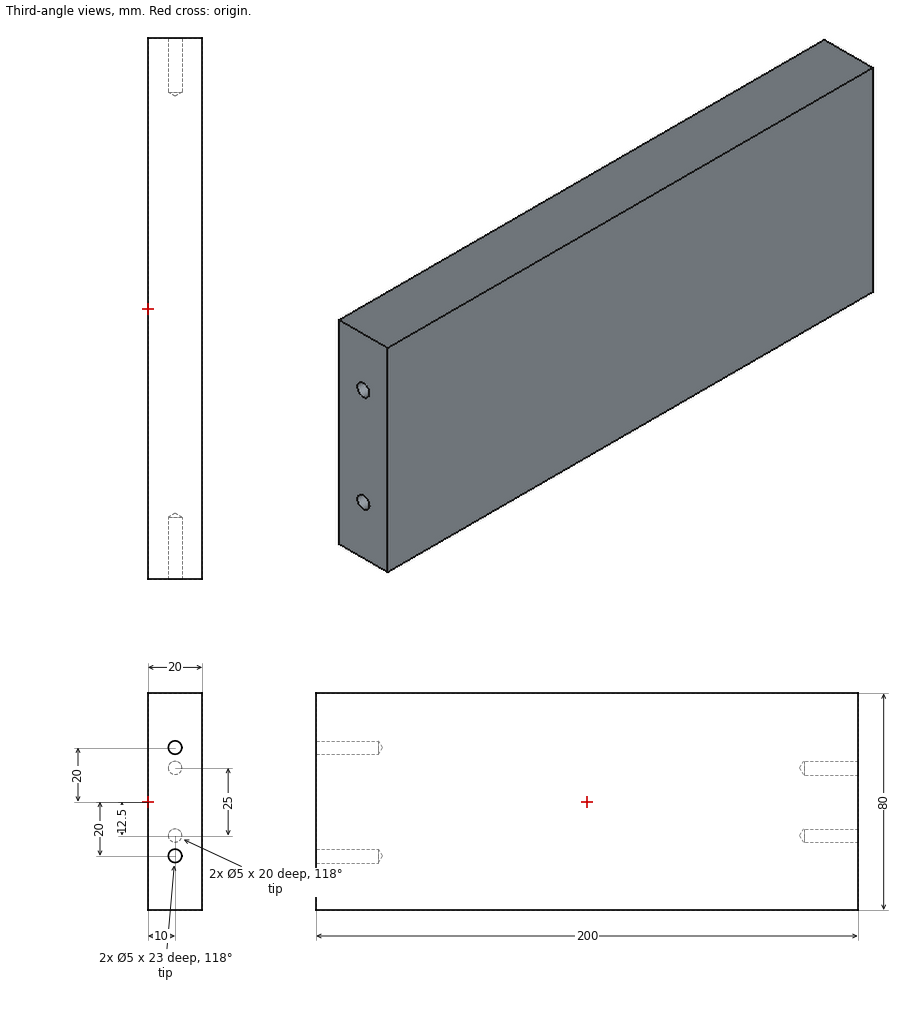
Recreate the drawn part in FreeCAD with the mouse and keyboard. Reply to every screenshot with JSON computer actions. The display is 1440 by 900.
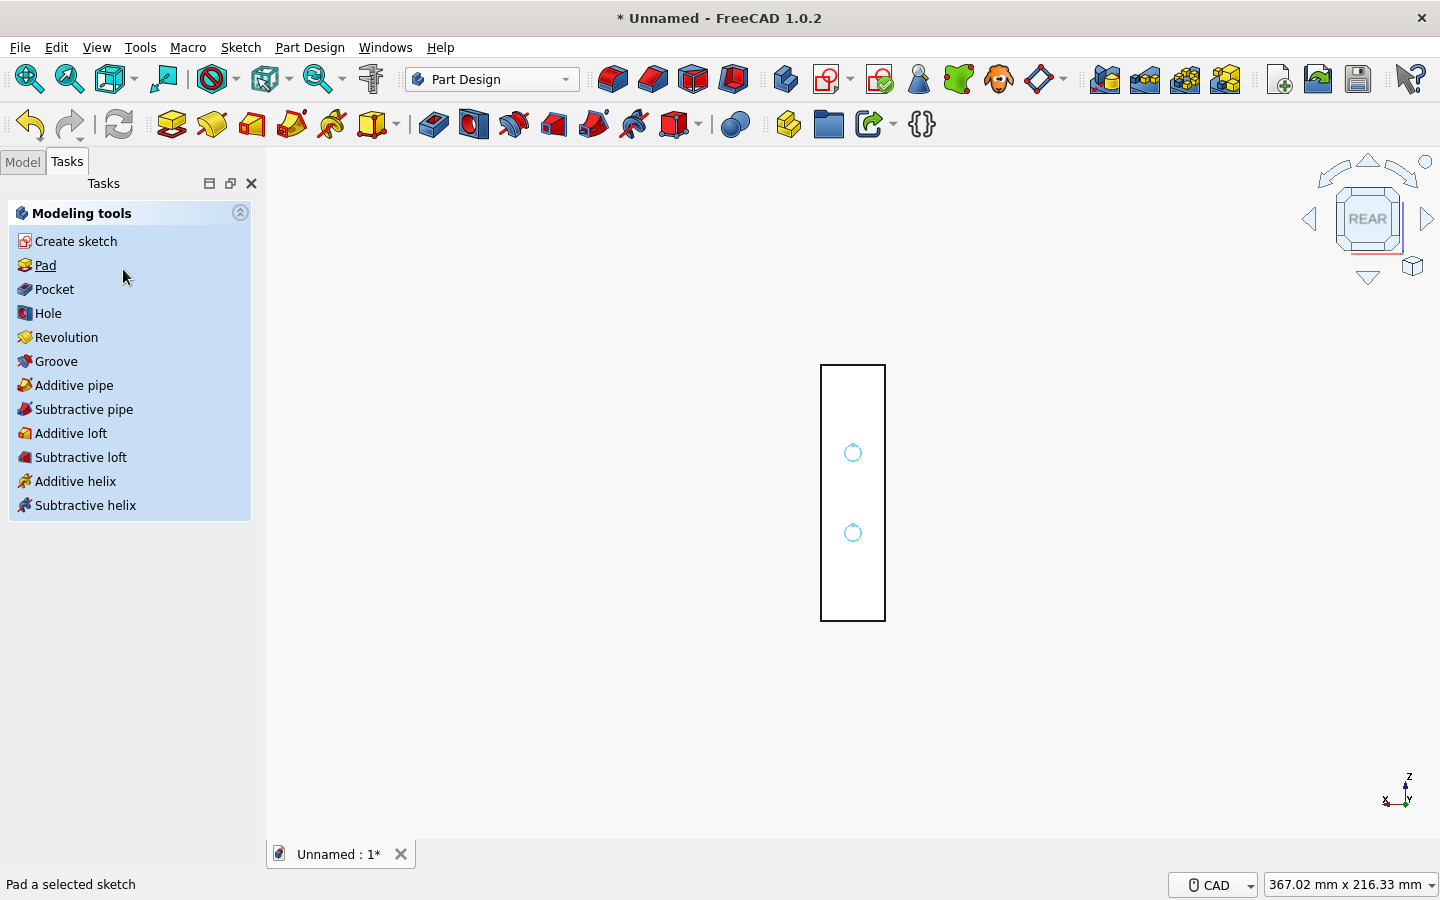
{"action": "left_click", "coordinate": [474, 124]}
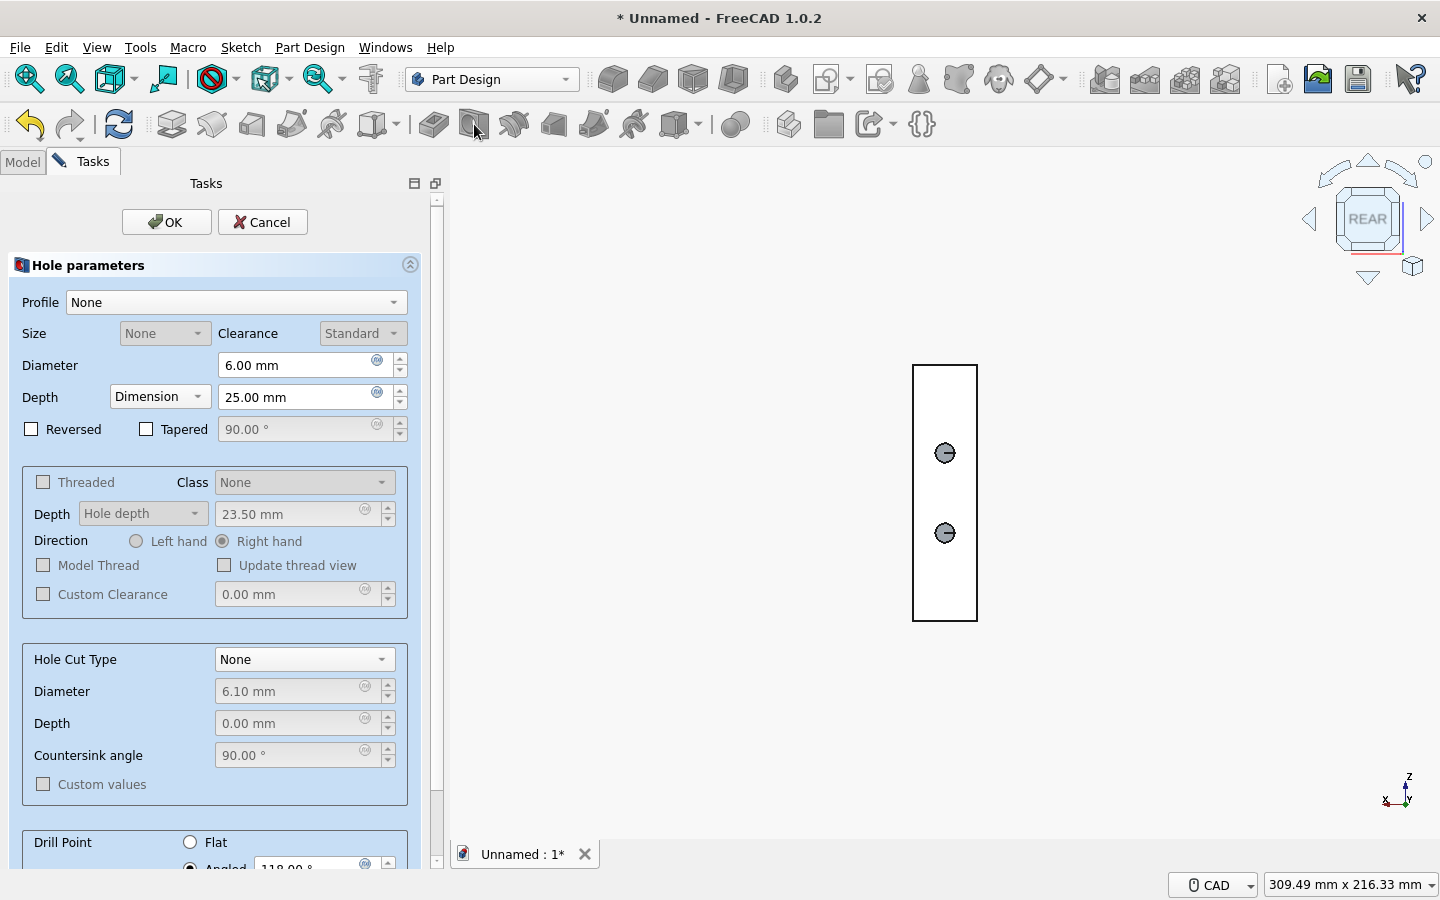
{"action": "triple_click", "coordinate": [305, 365]}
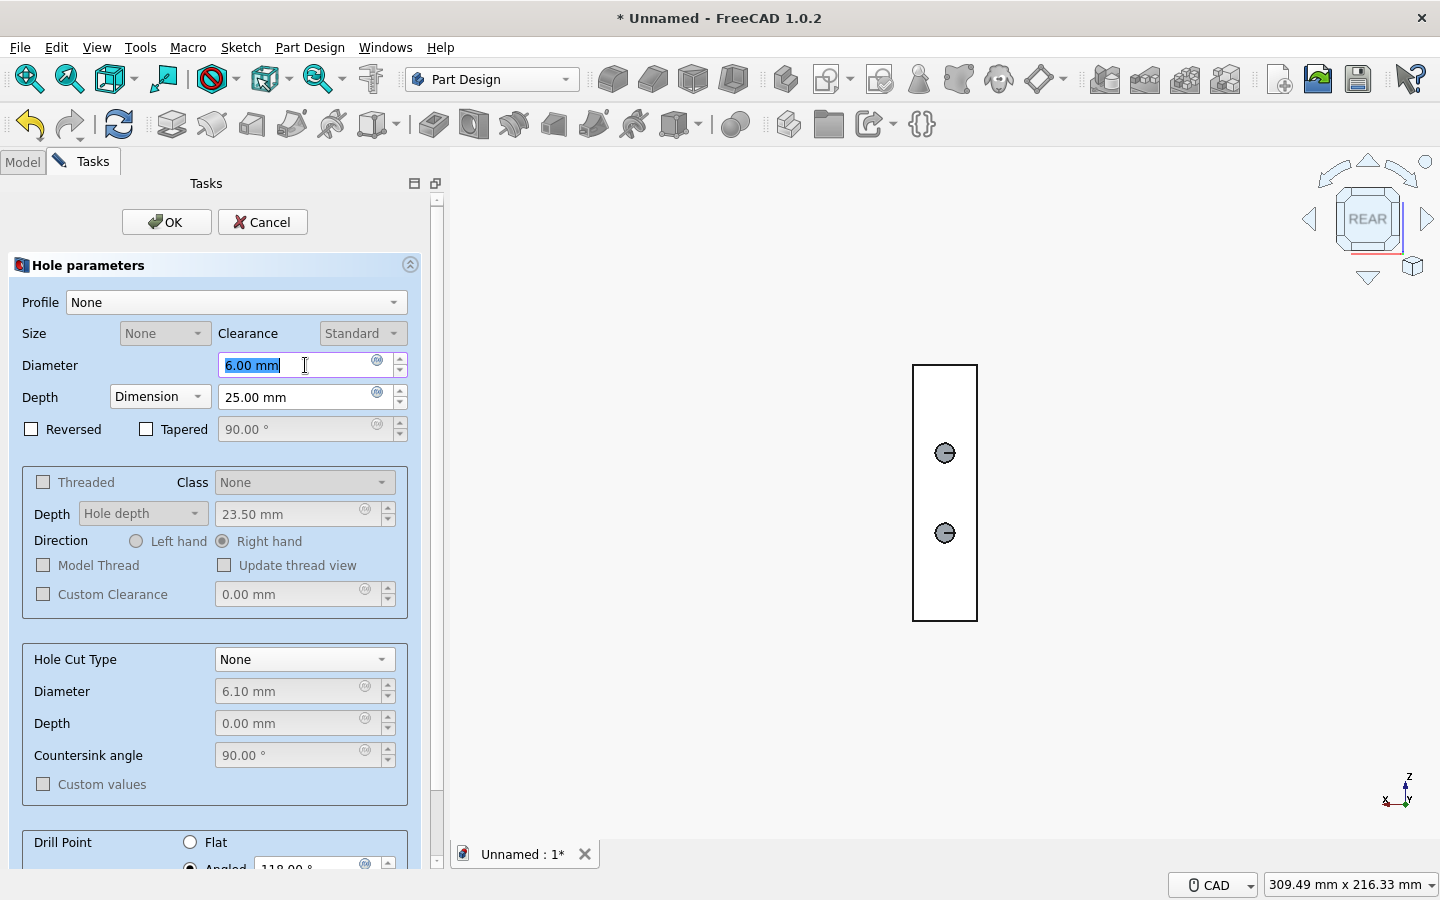
{"action": "type", "text": "5"}
{"action": "key", "text": "Tab"}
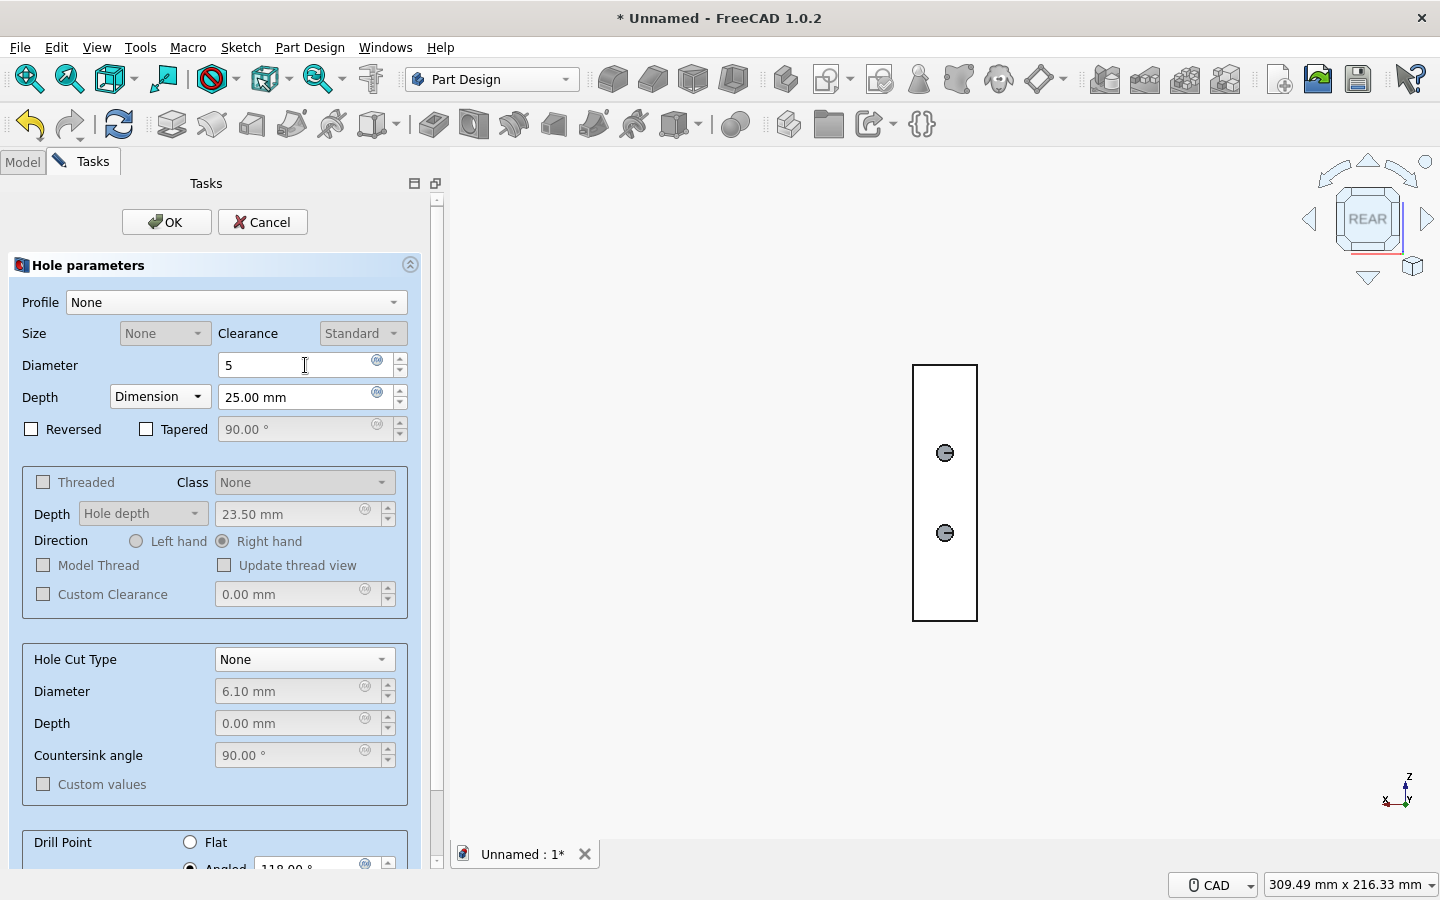
{"action": "triple_click", "coordinate": [305, 397]}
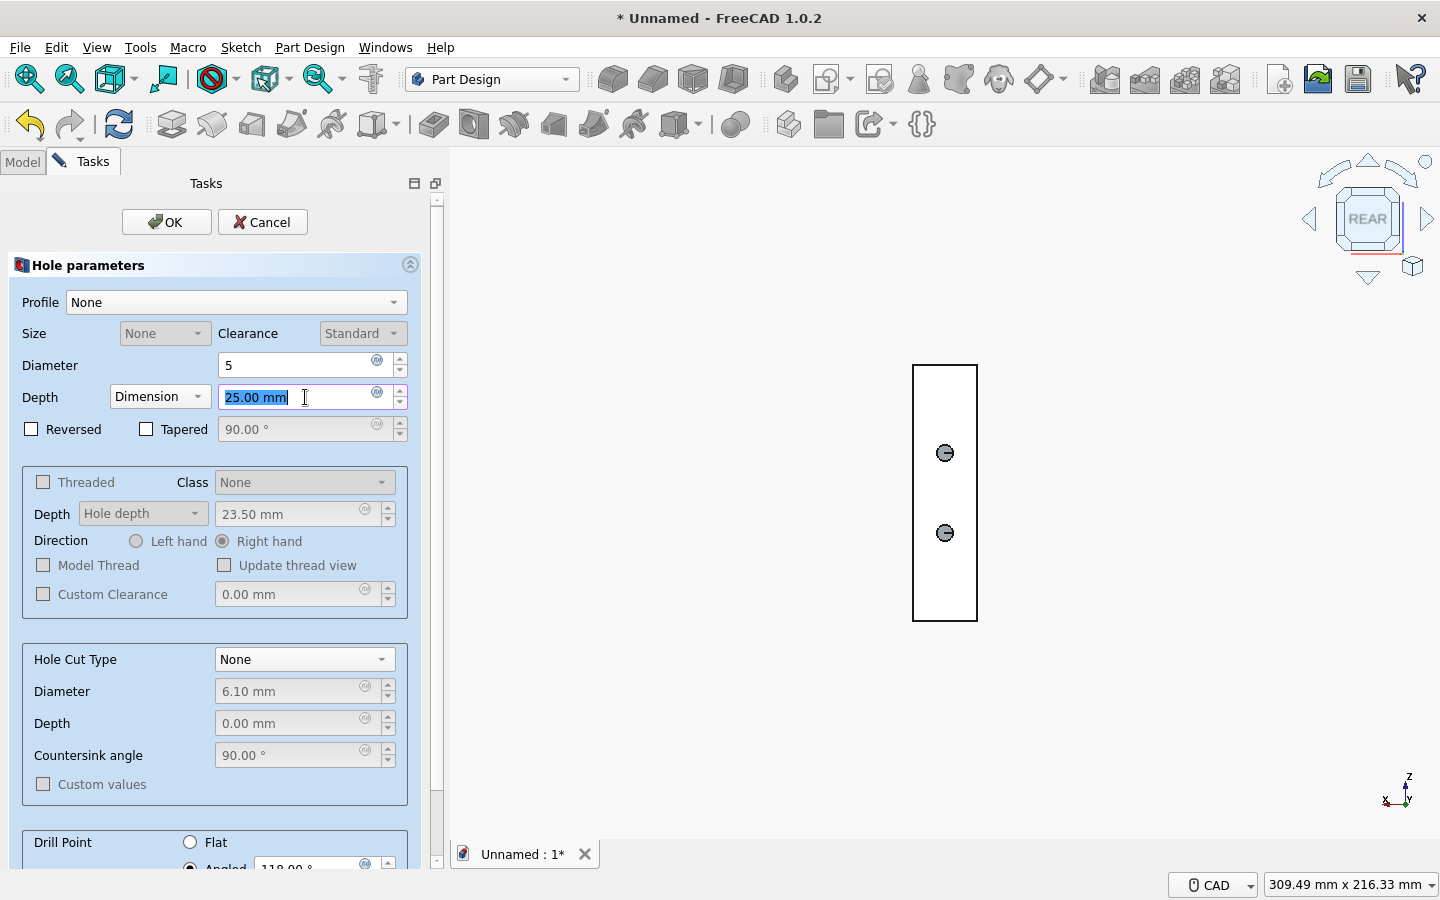
{"action": "type", "text": "20"}
{"action": "key", "text": "Tab"}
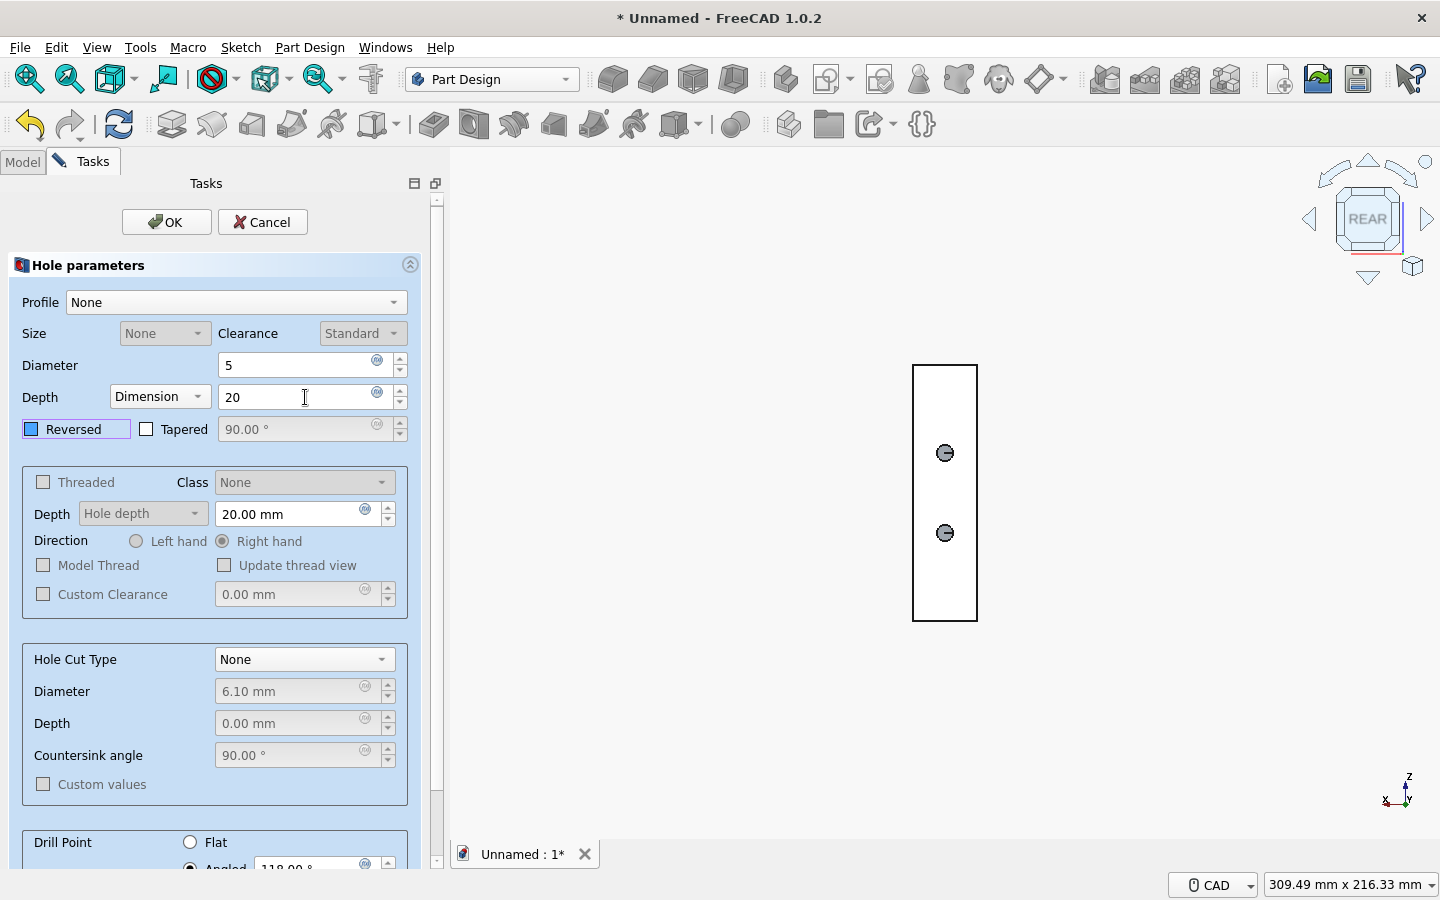
{"action": "left_click", "coordinate": [167, 222]}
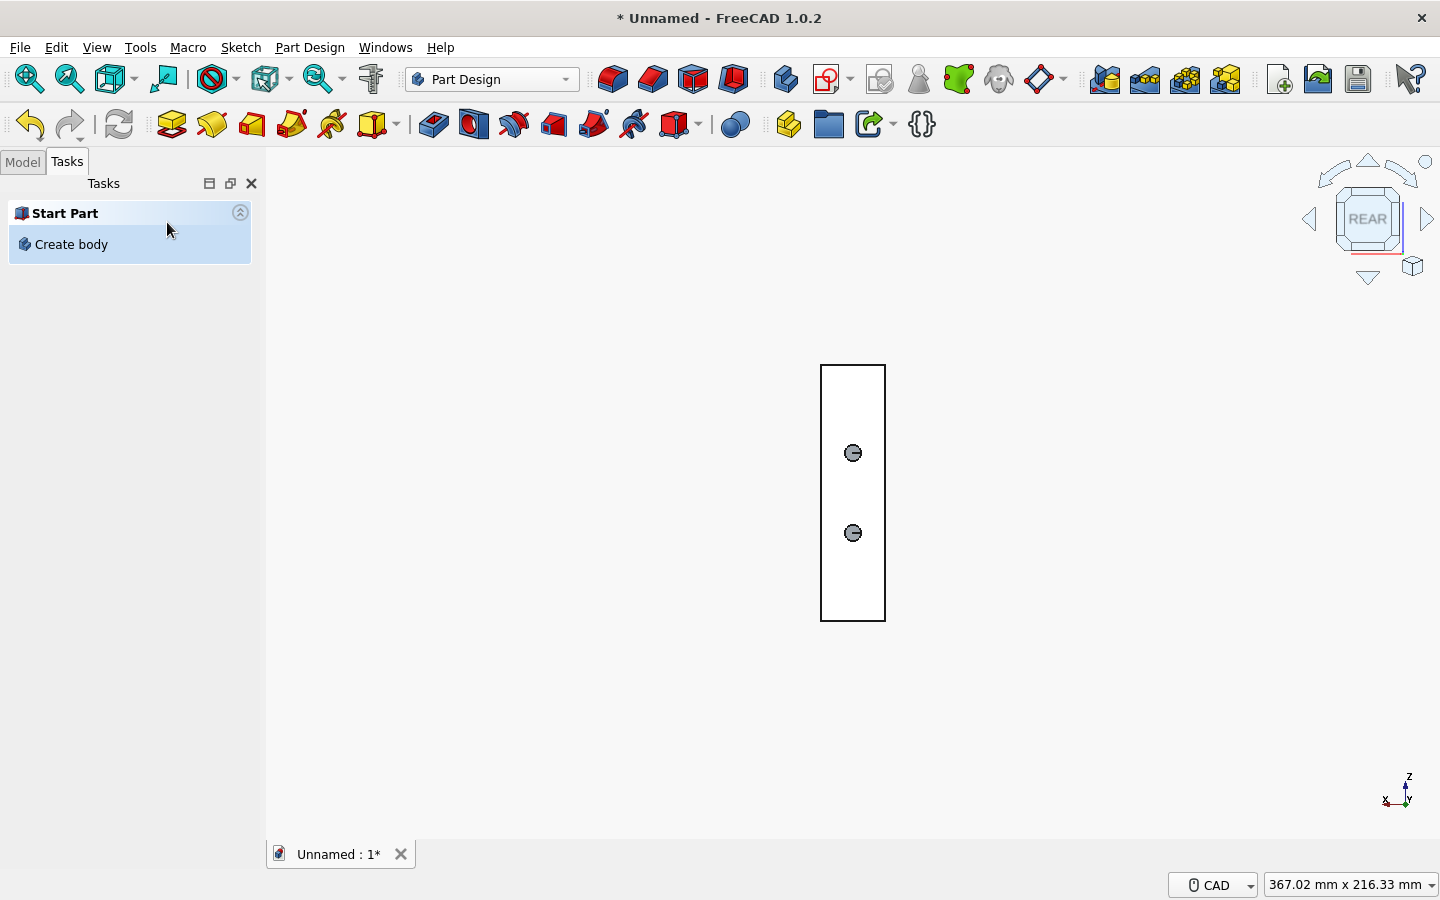
{"action": "key", "text": "v f"}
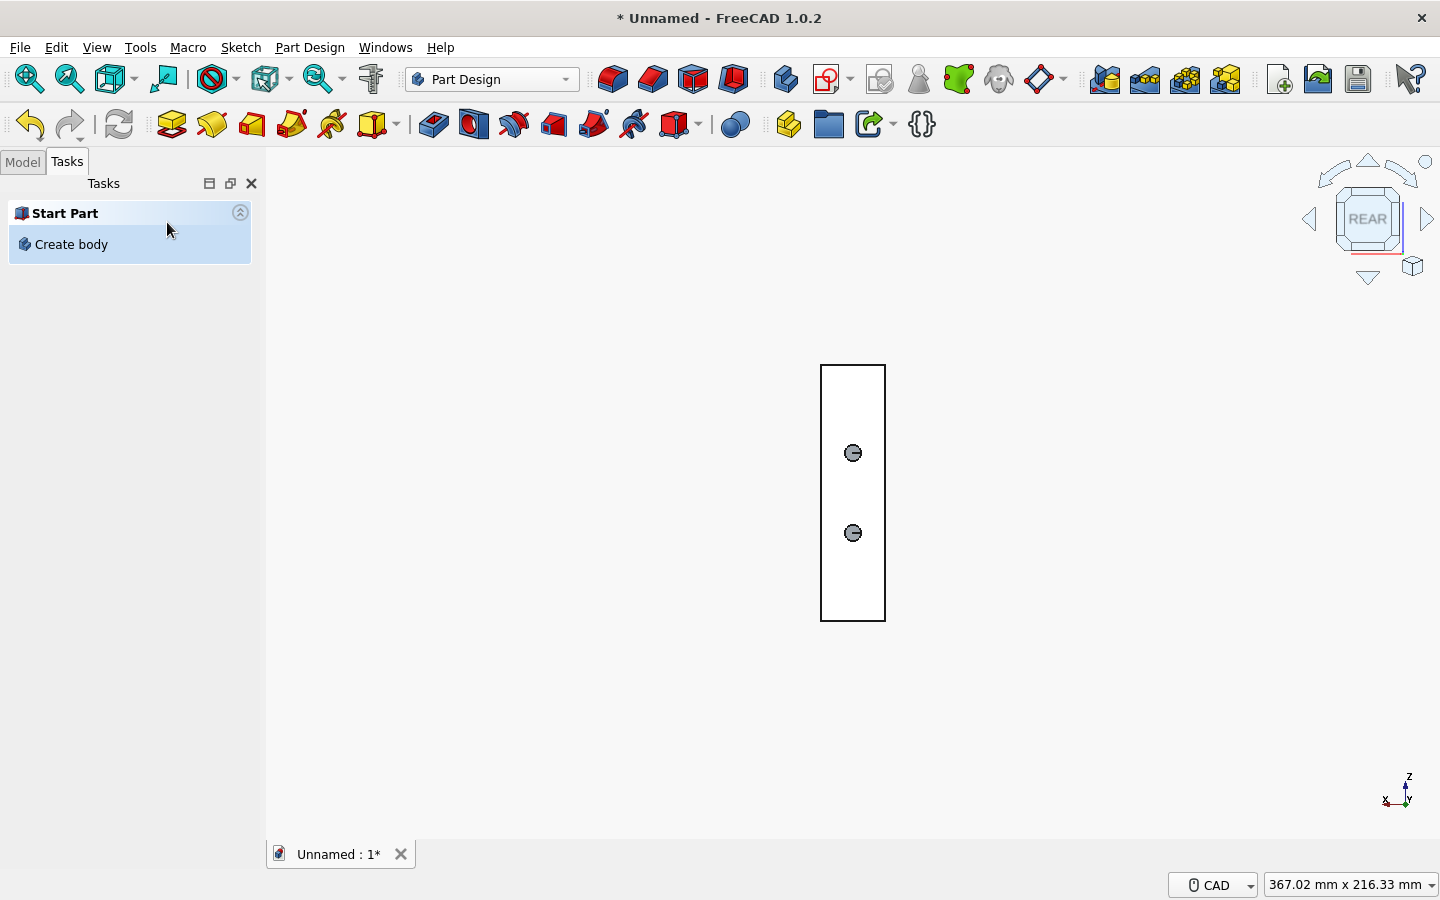
{"action": "key", "text": "0"}